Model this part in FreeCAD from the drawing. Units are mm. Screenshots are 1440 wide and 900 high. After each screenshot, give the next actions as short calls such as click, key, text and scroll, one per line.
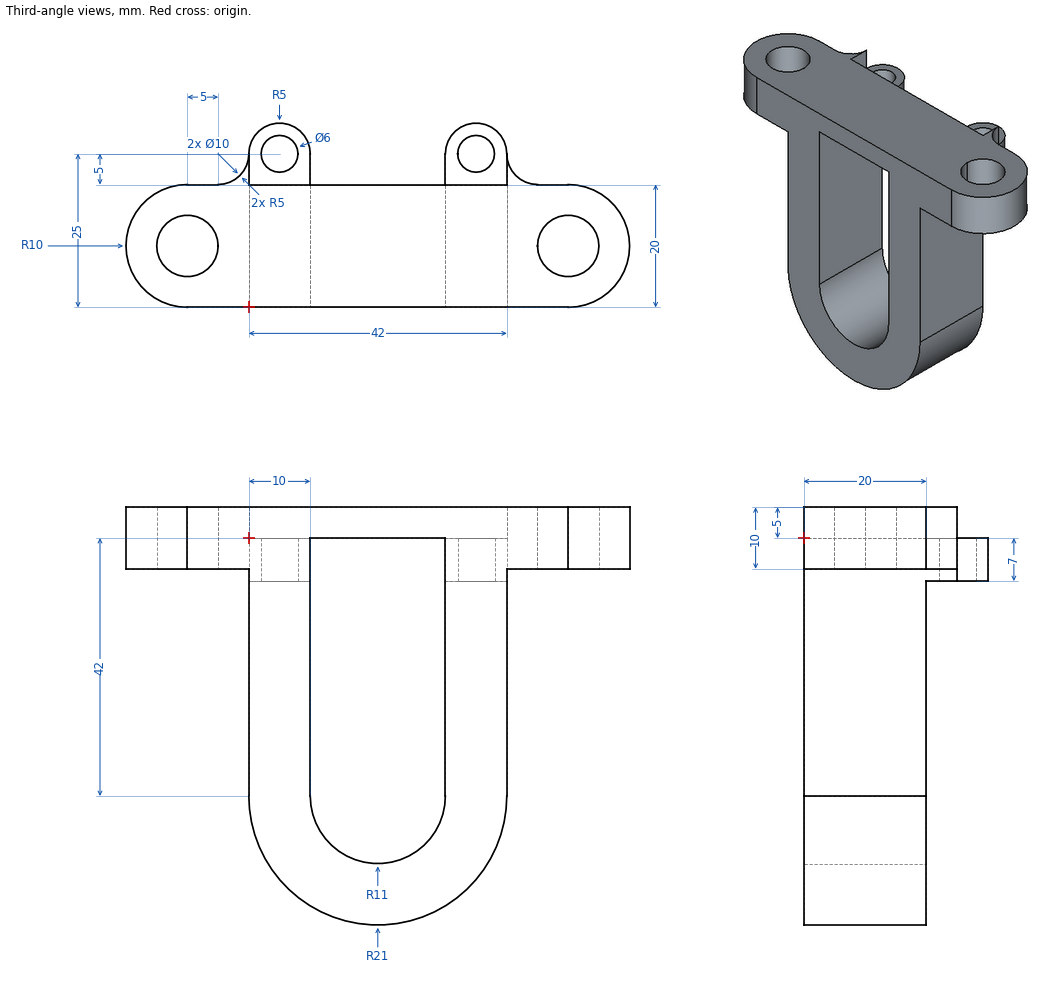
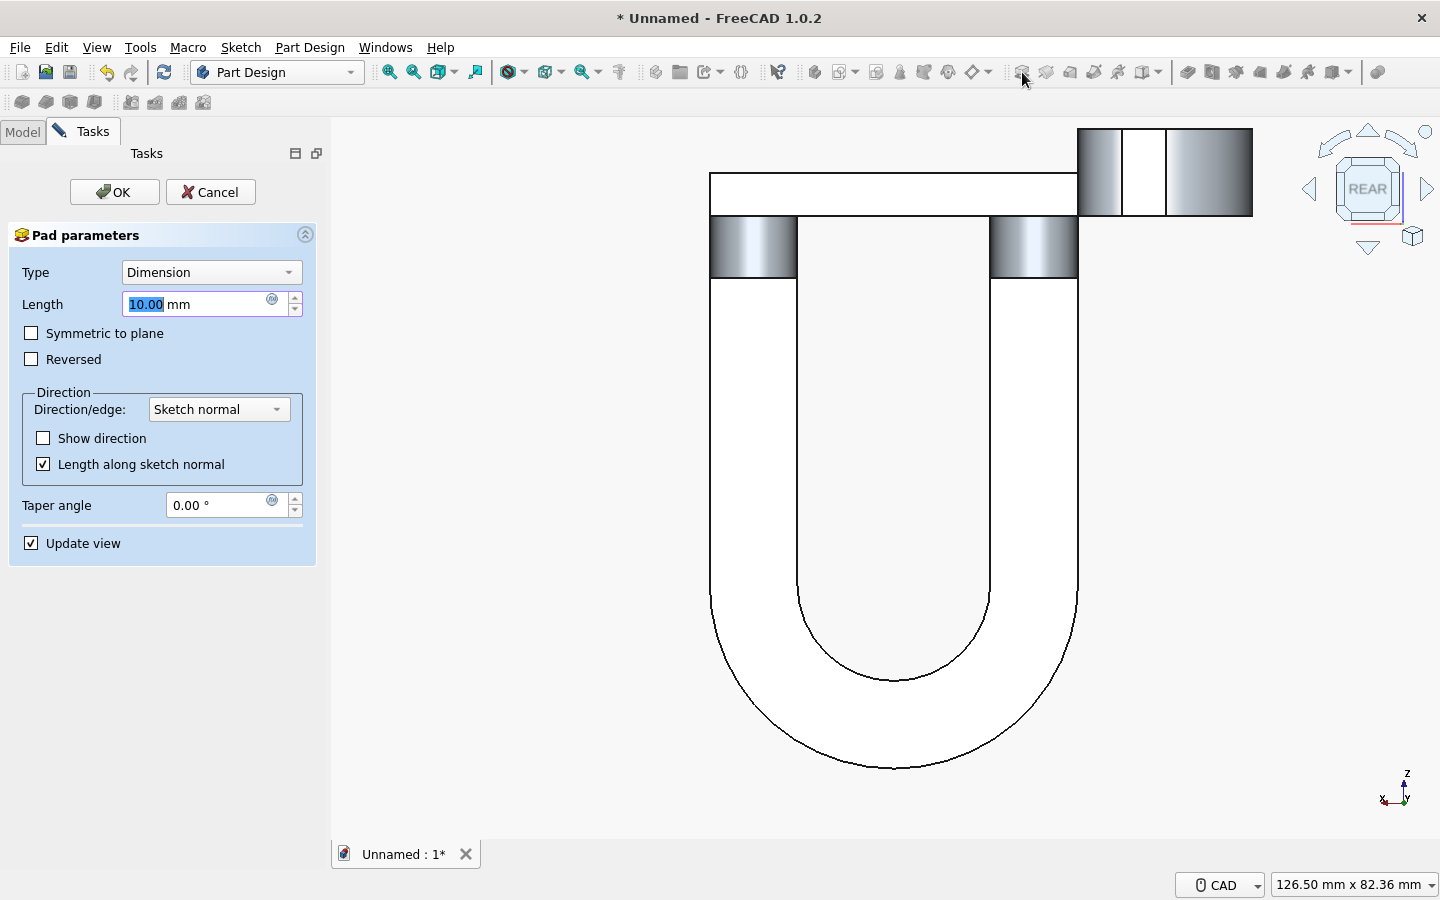
text(10)
key(Tab)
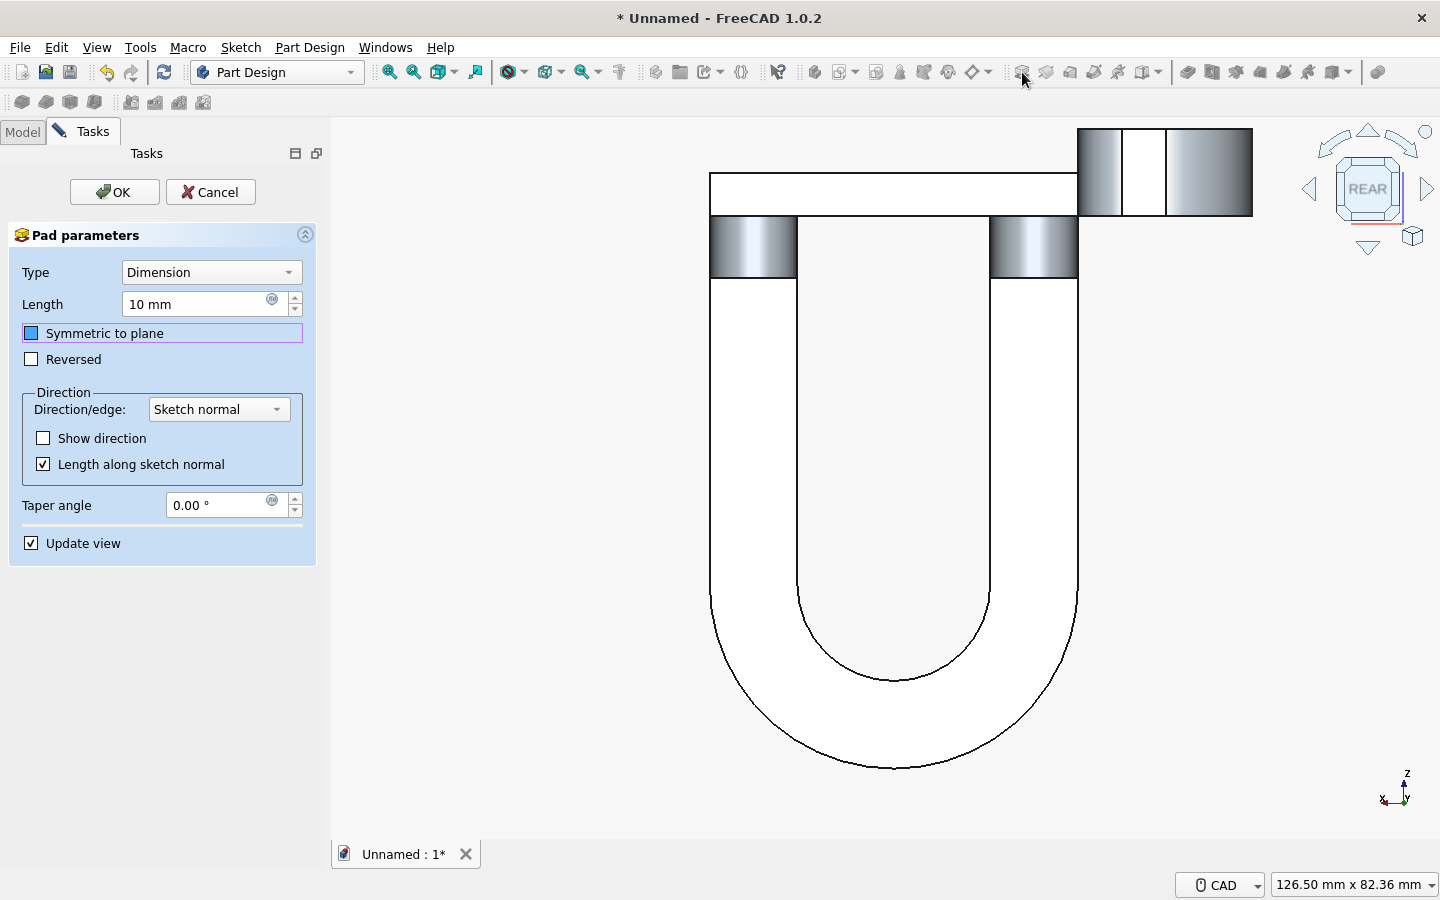
click(30, 333)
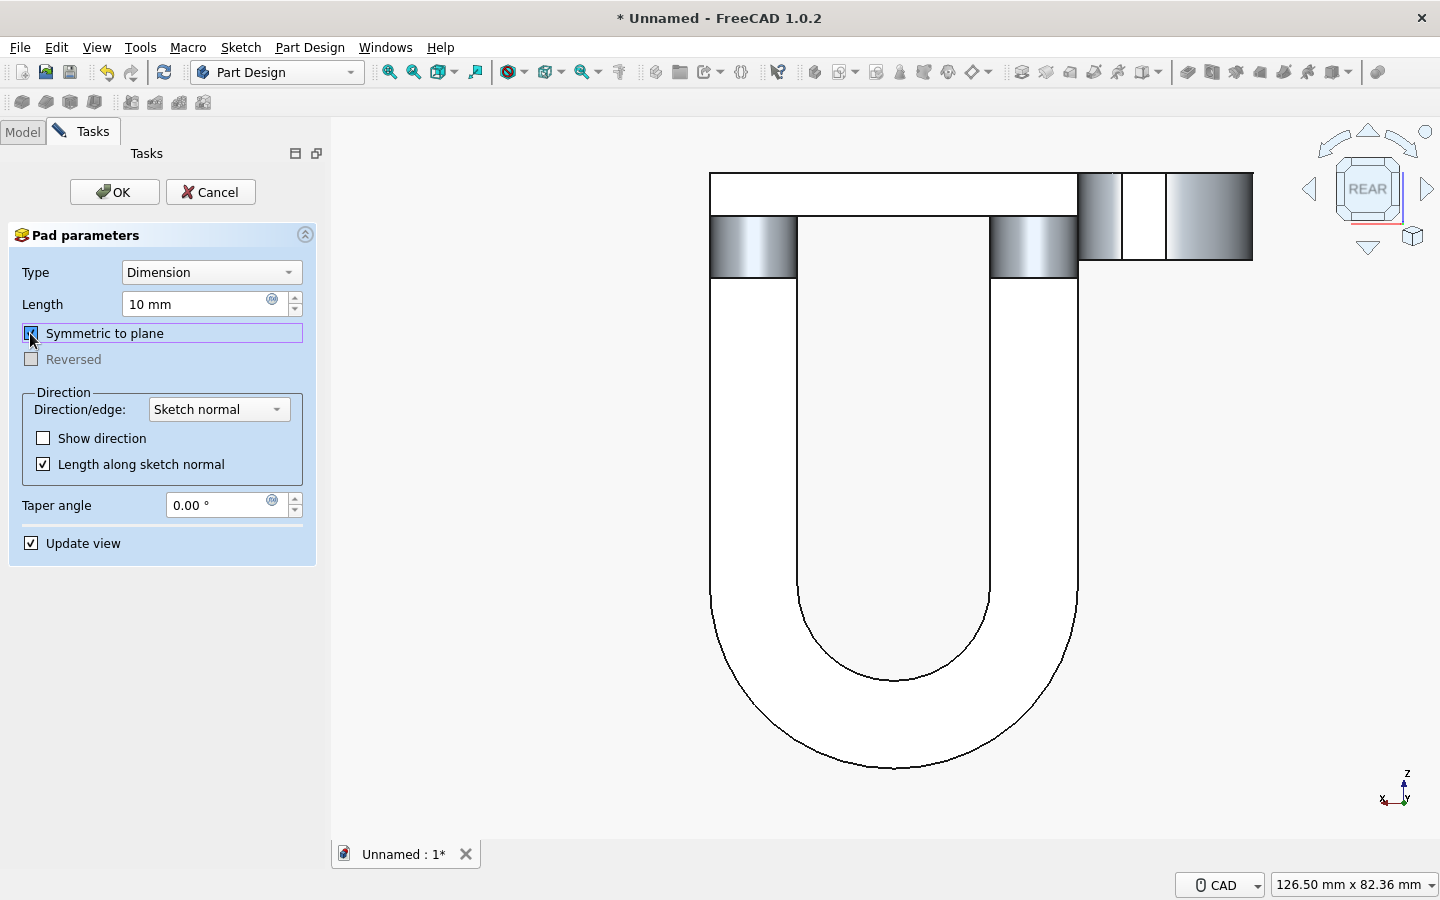
click(115, 192)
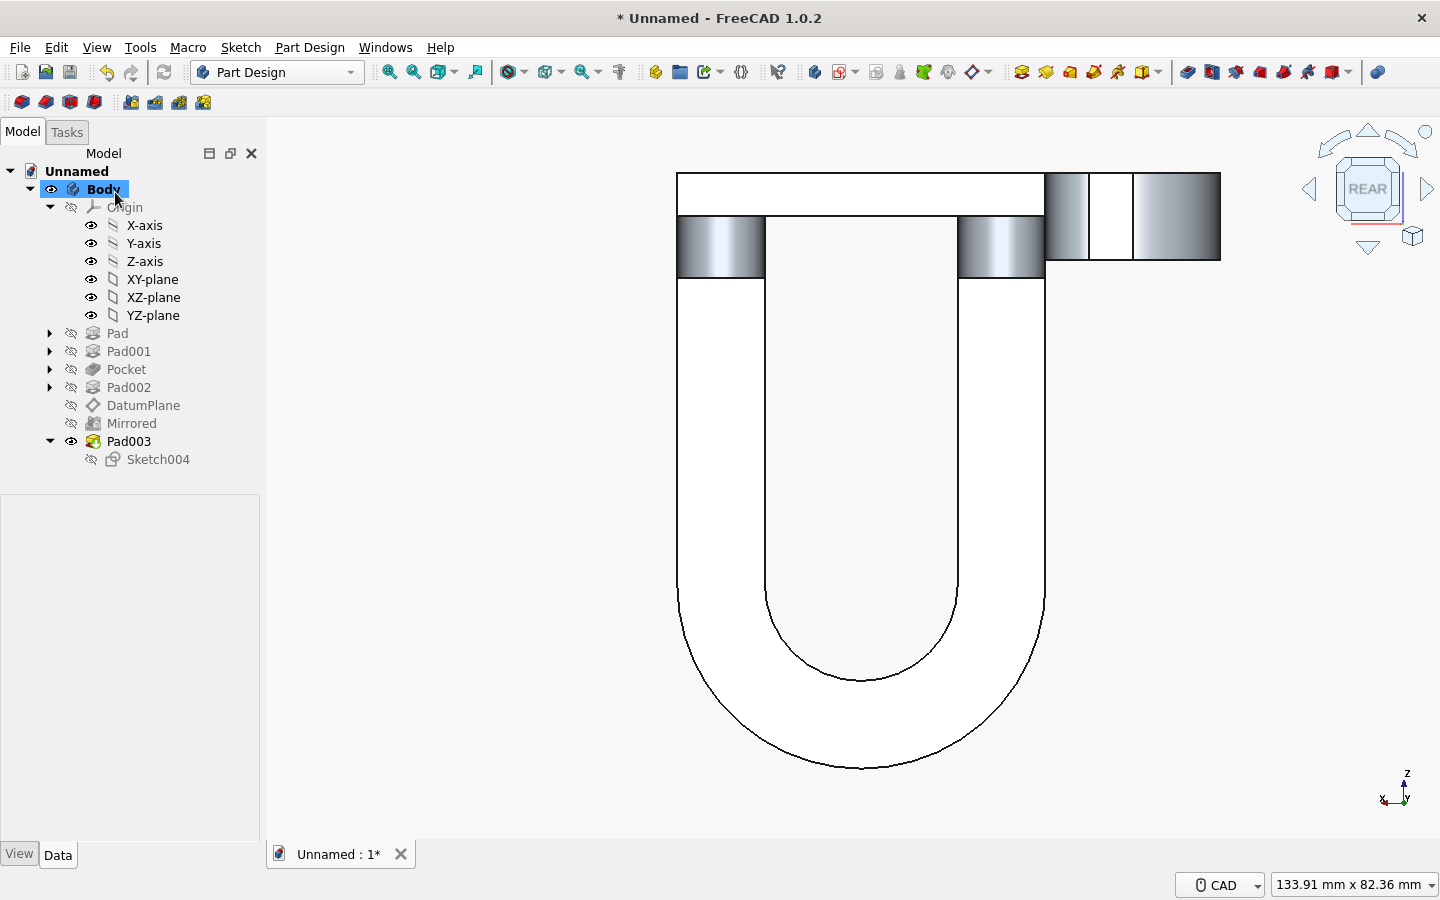
click(136, 315)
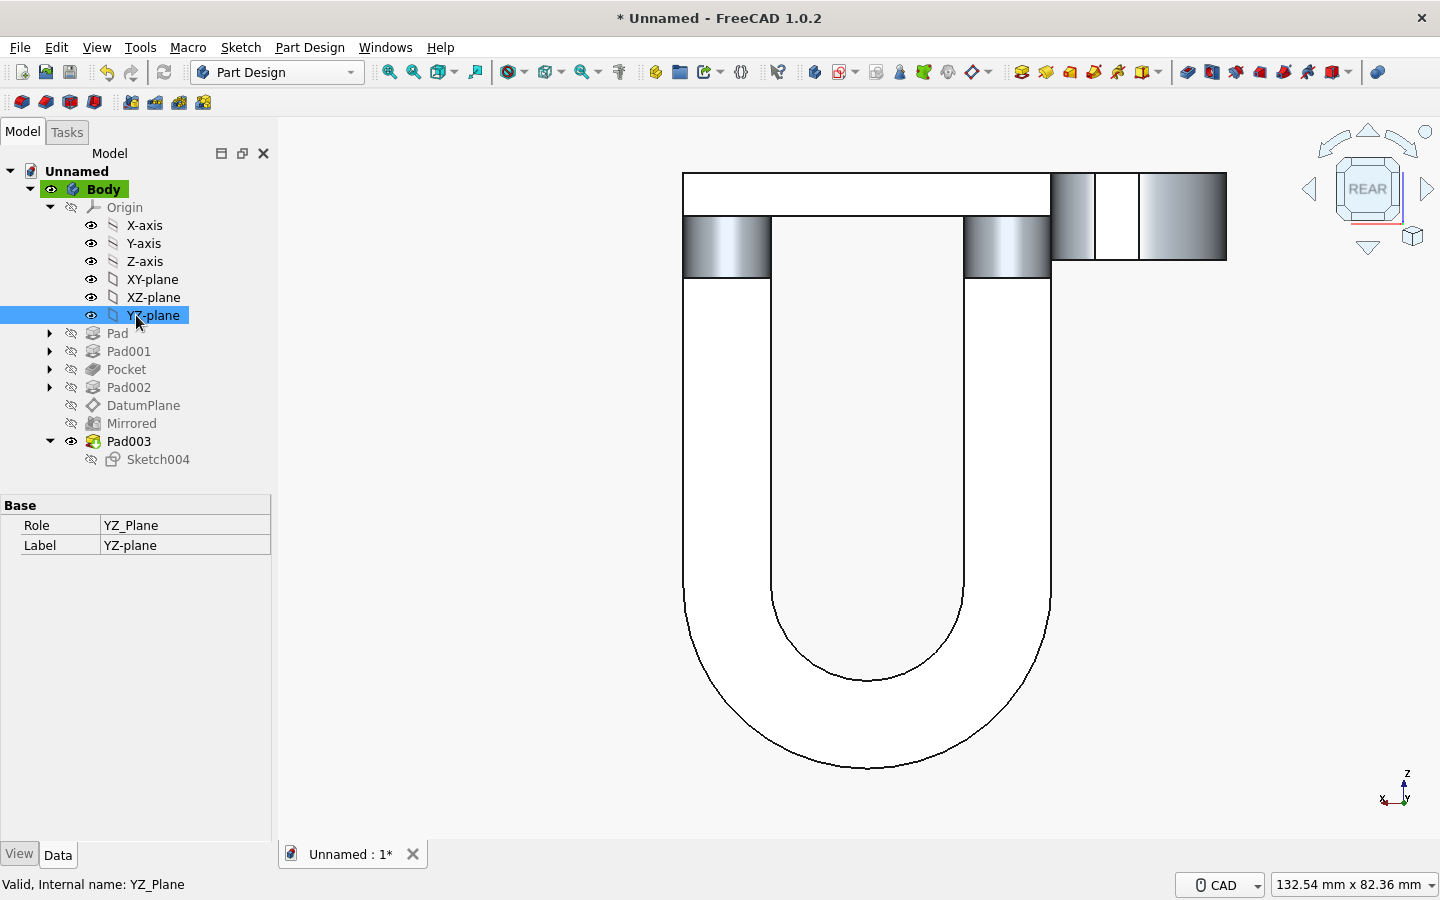
click(972, 72)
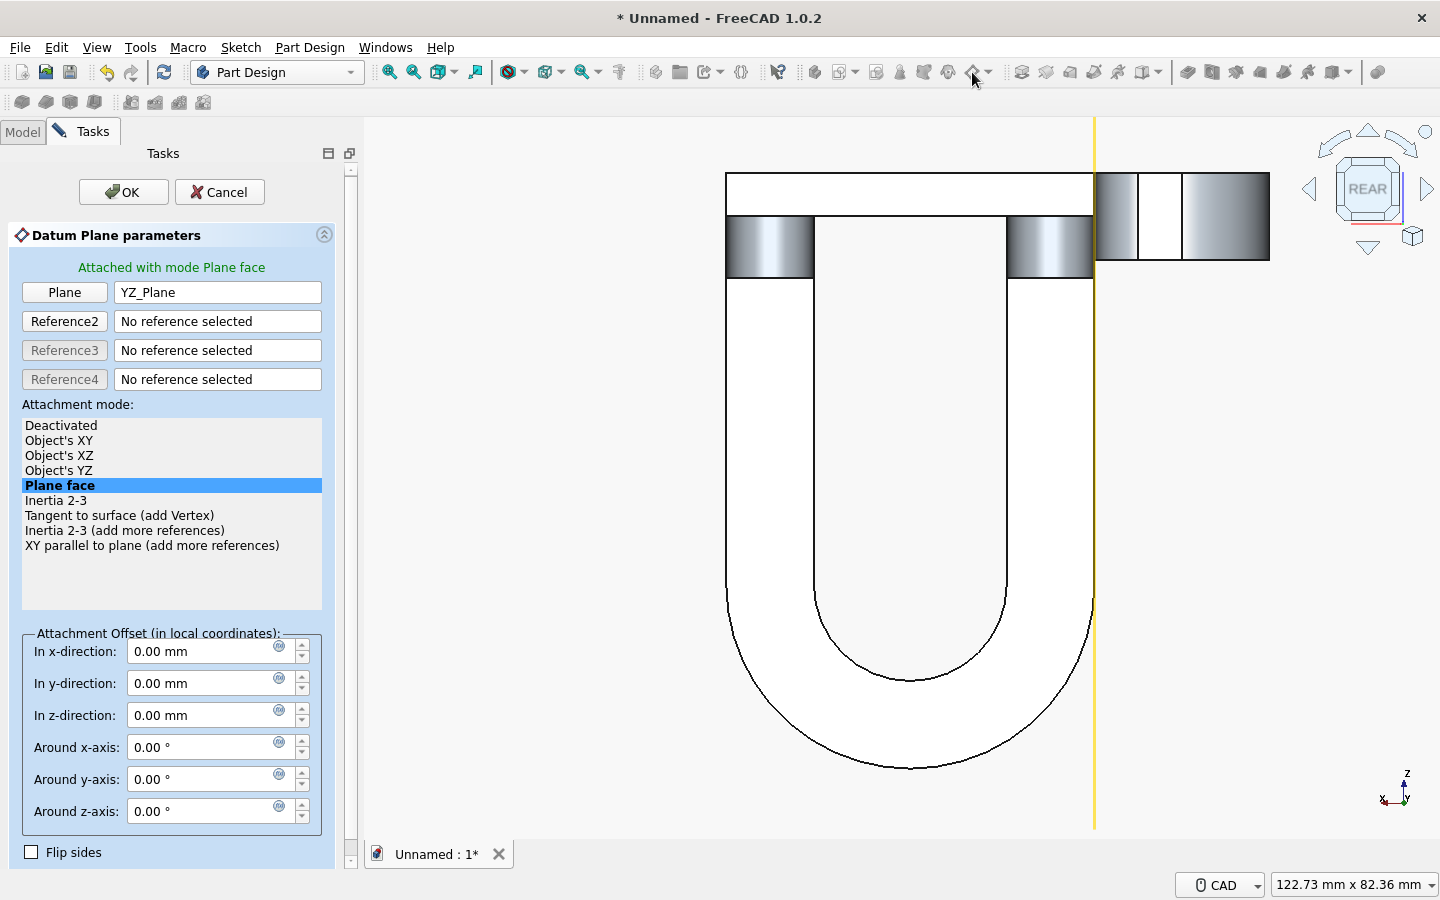
triple_click(210, 715)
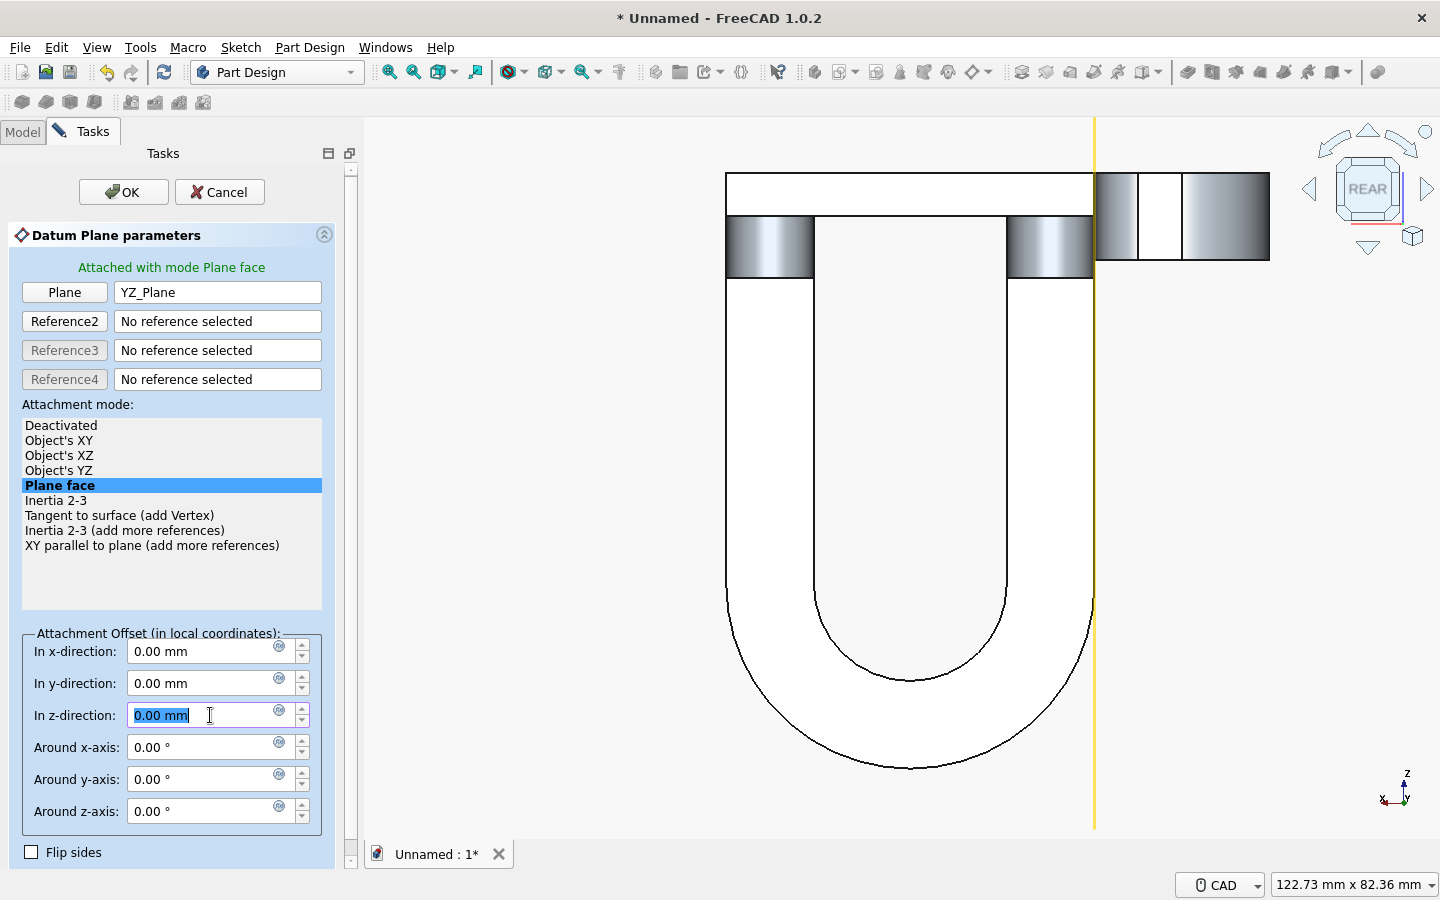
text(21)
key(Tab)